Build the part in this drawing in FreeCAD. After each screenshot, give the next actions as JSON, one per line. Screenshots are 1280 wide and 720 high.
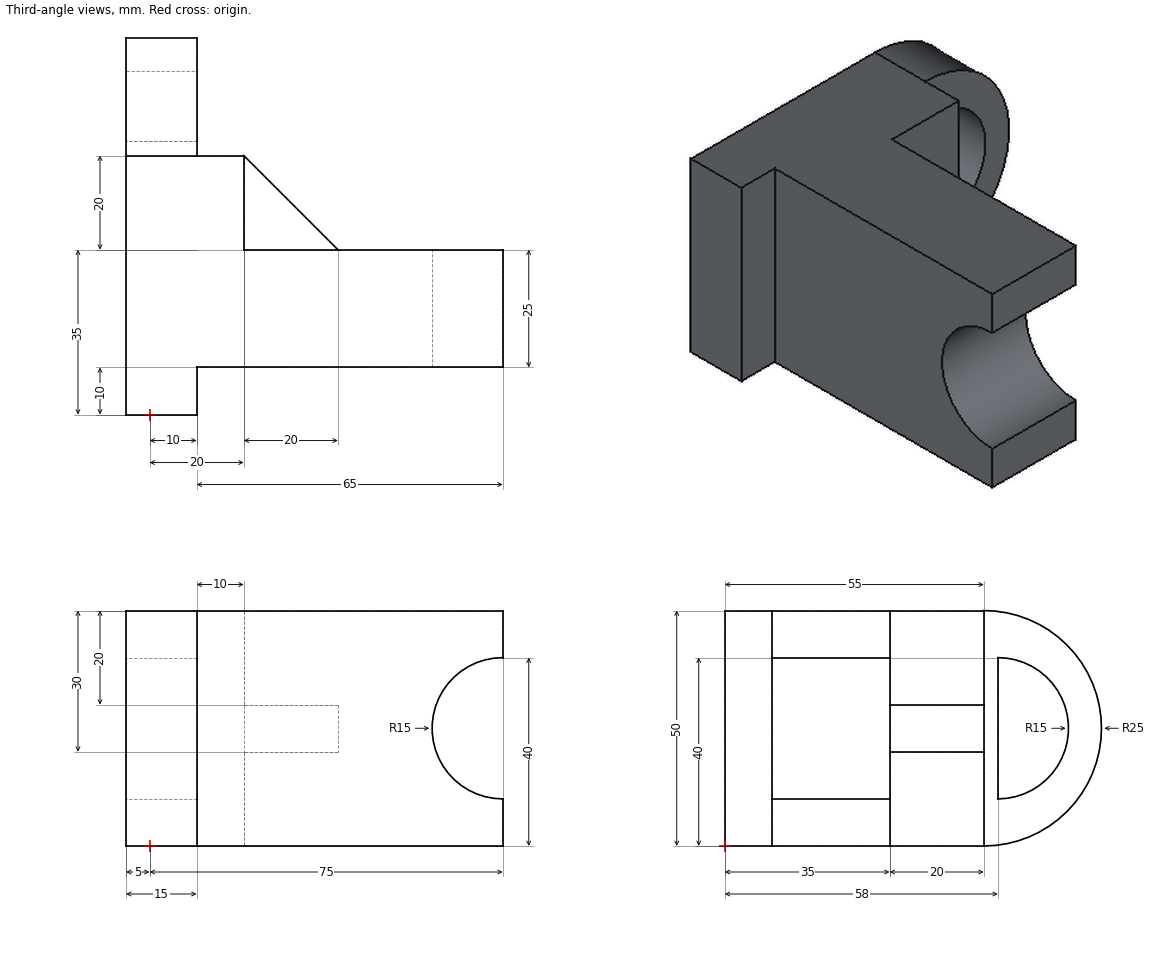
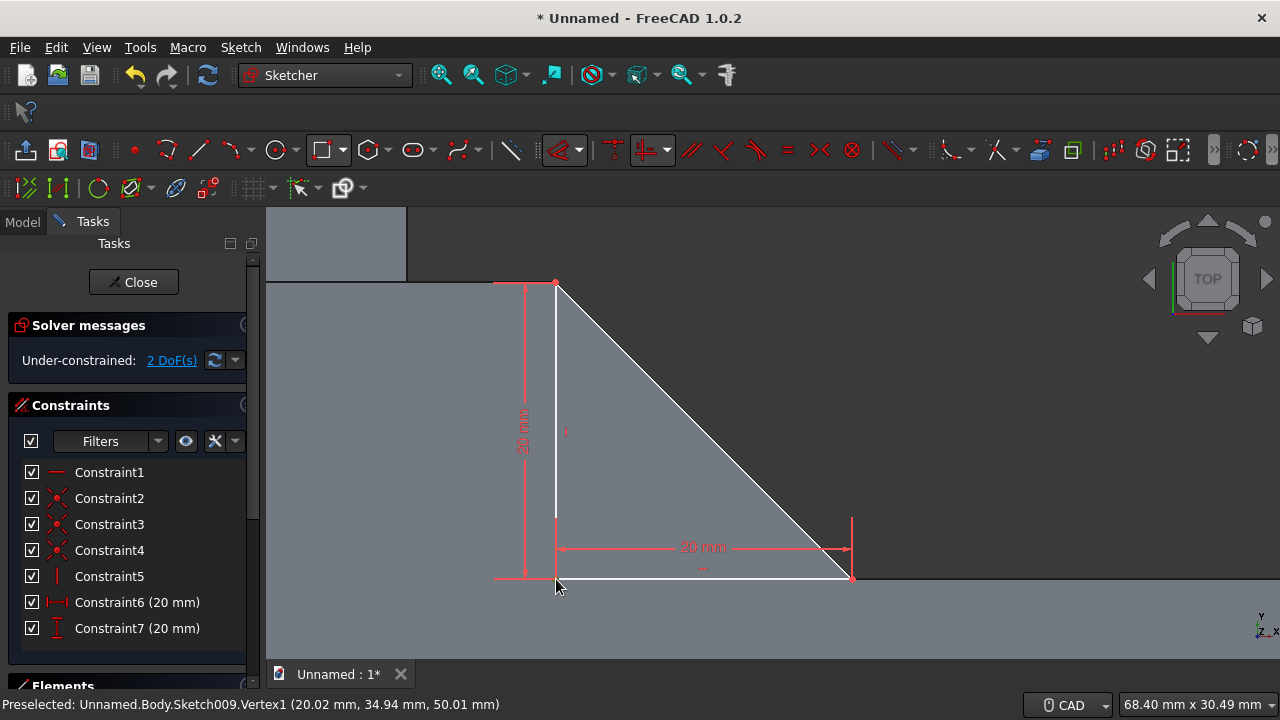
{"action": "key", "text": "l"}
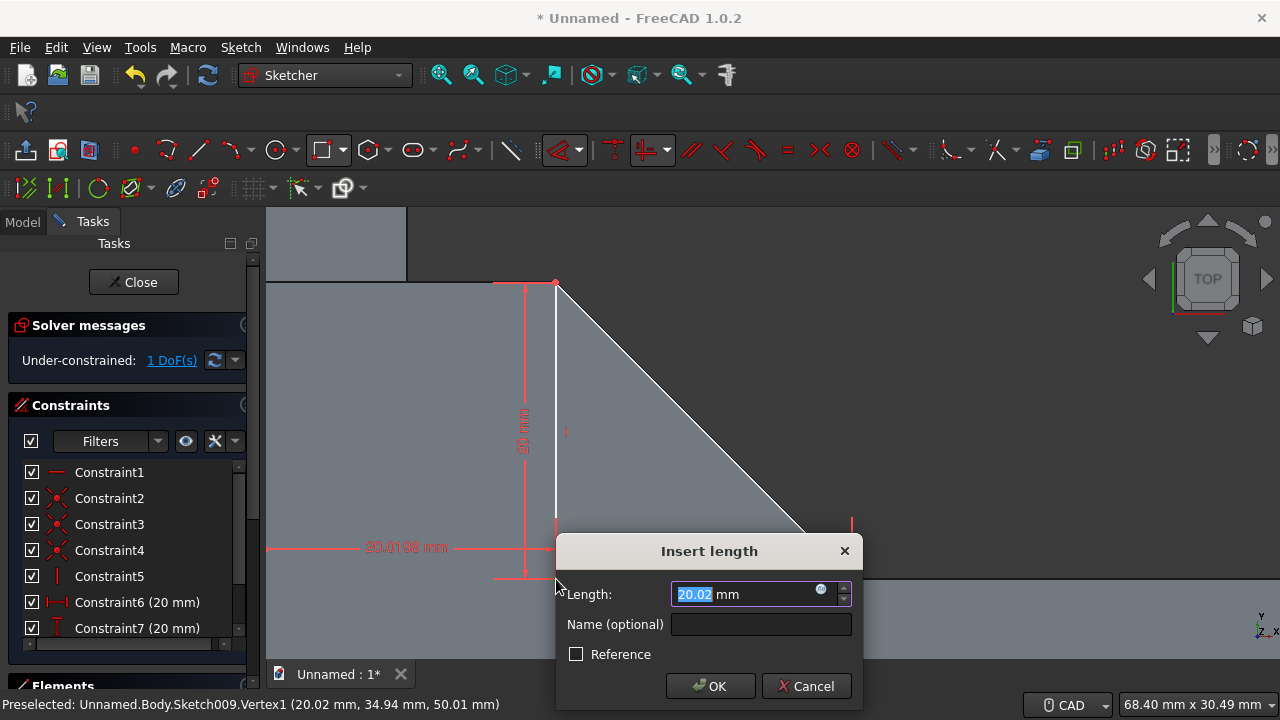
{"action": "type", "text": "20"}
{"action": "key", "text": "Return"}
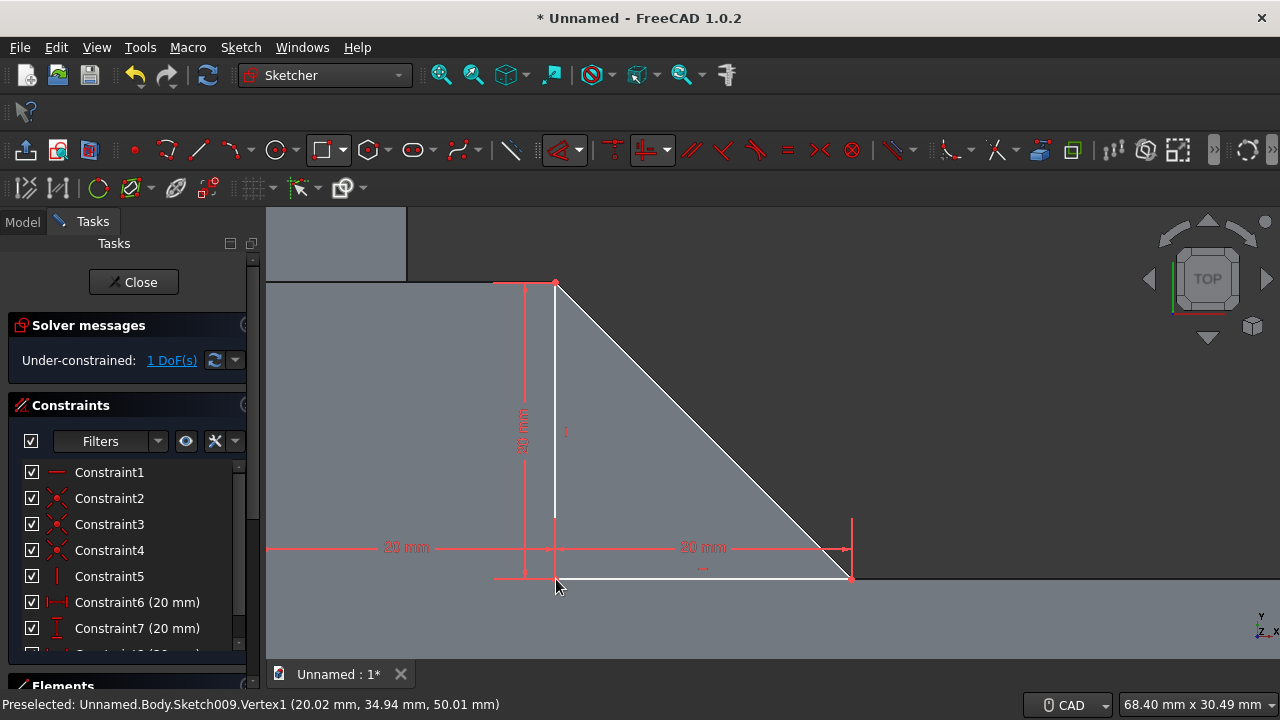
{"action": "left_click", "coordinate": [555, 579]}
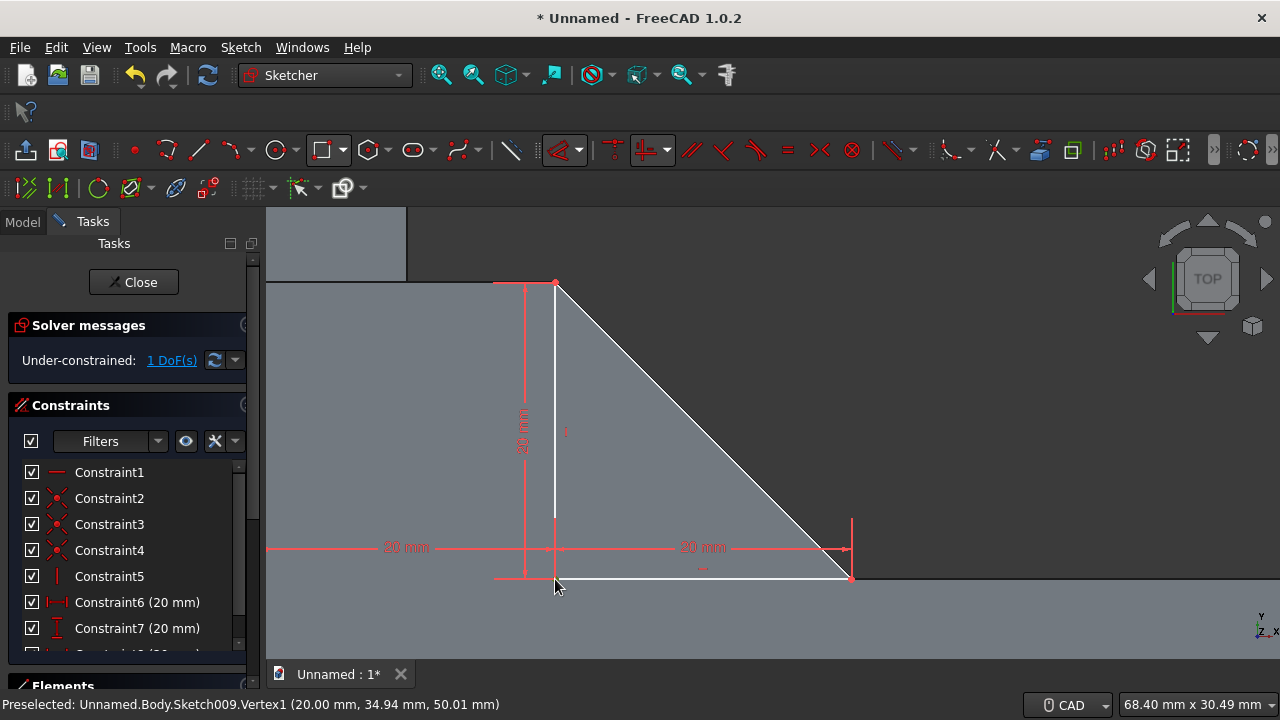
{"action": "left_click", "coordinate": [582, 150]}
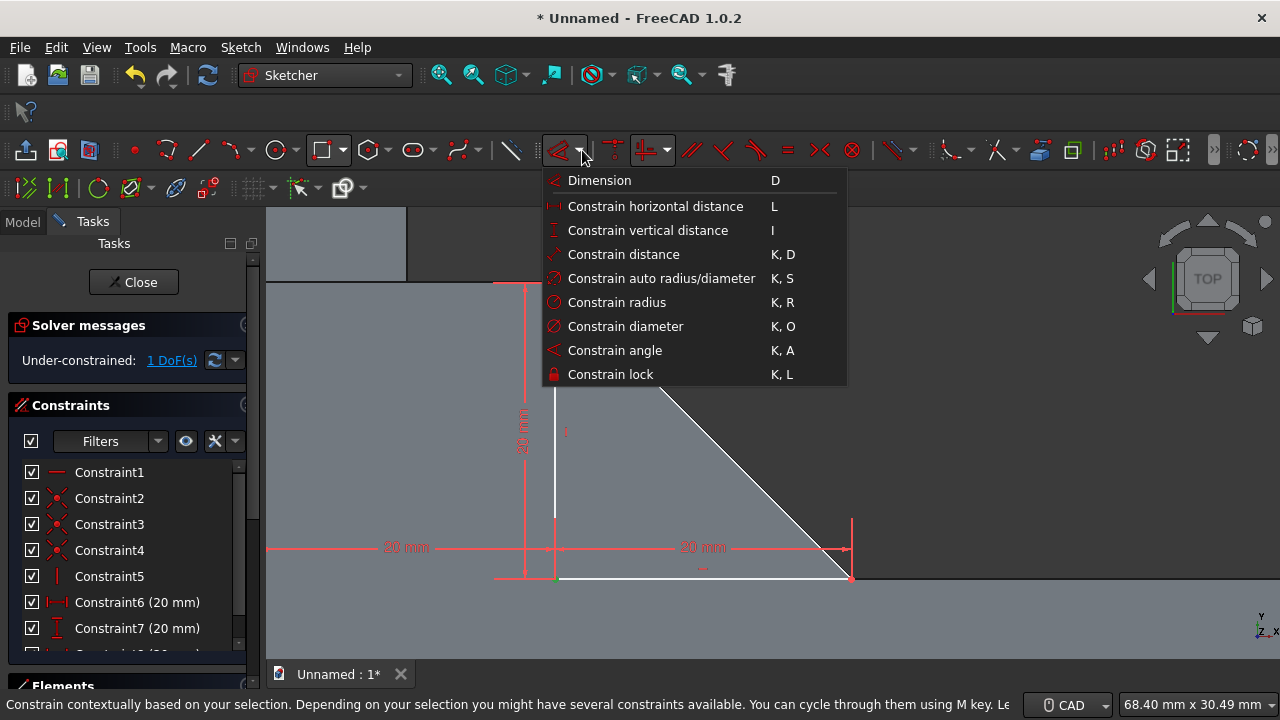
{"action": "left_click", "coordinate": [695, 230]}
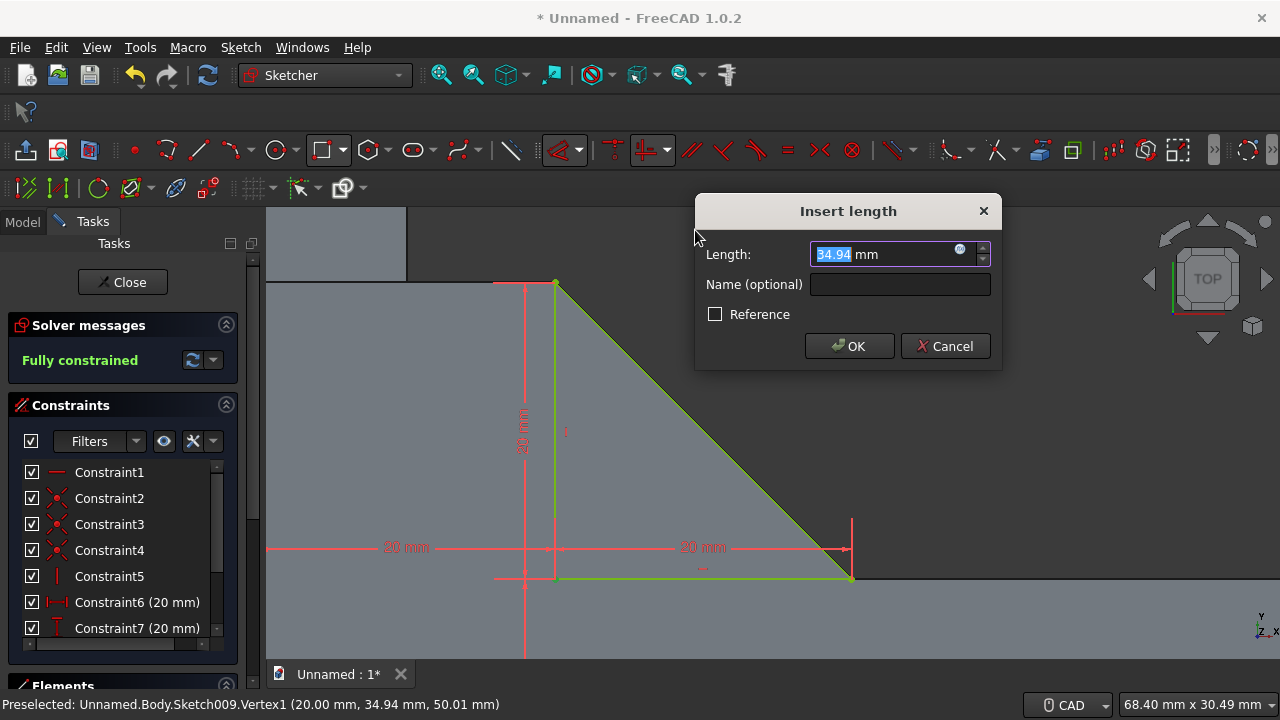
{"action": "type", "text": "35"}
{"action": "key", "text": "Return"}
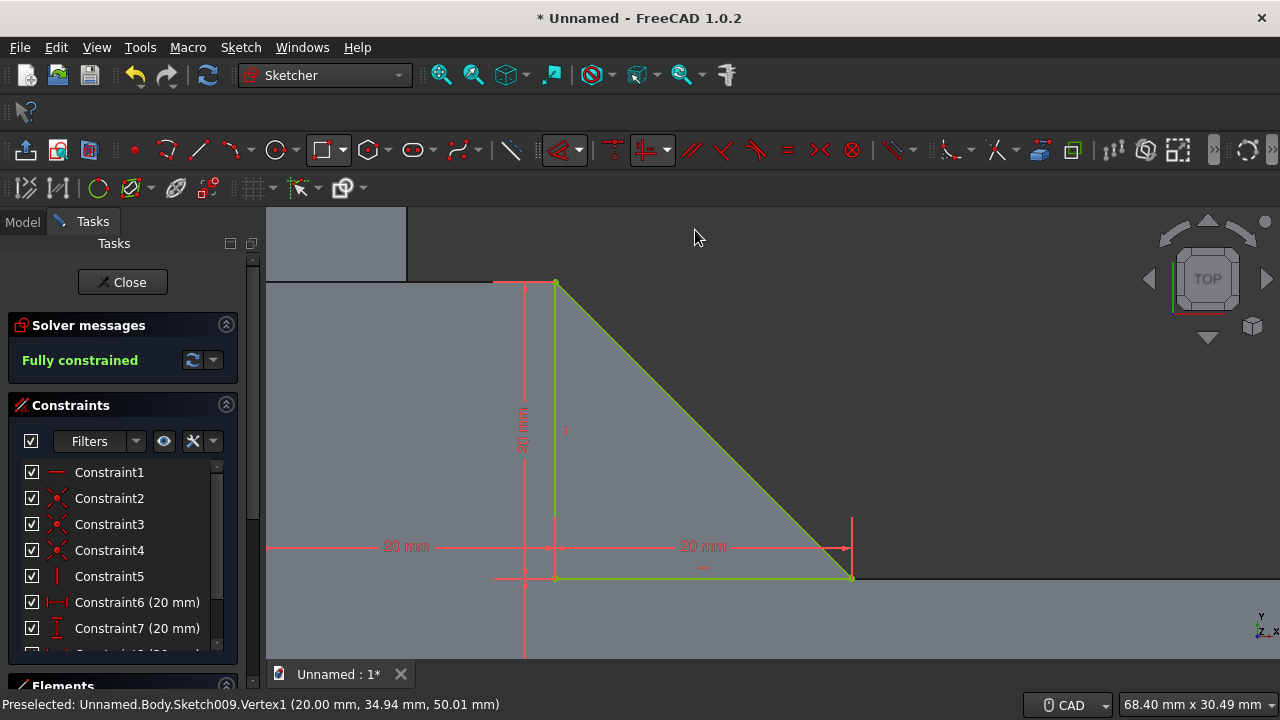
{"action": "left_click", "coordinate": [123, 282]}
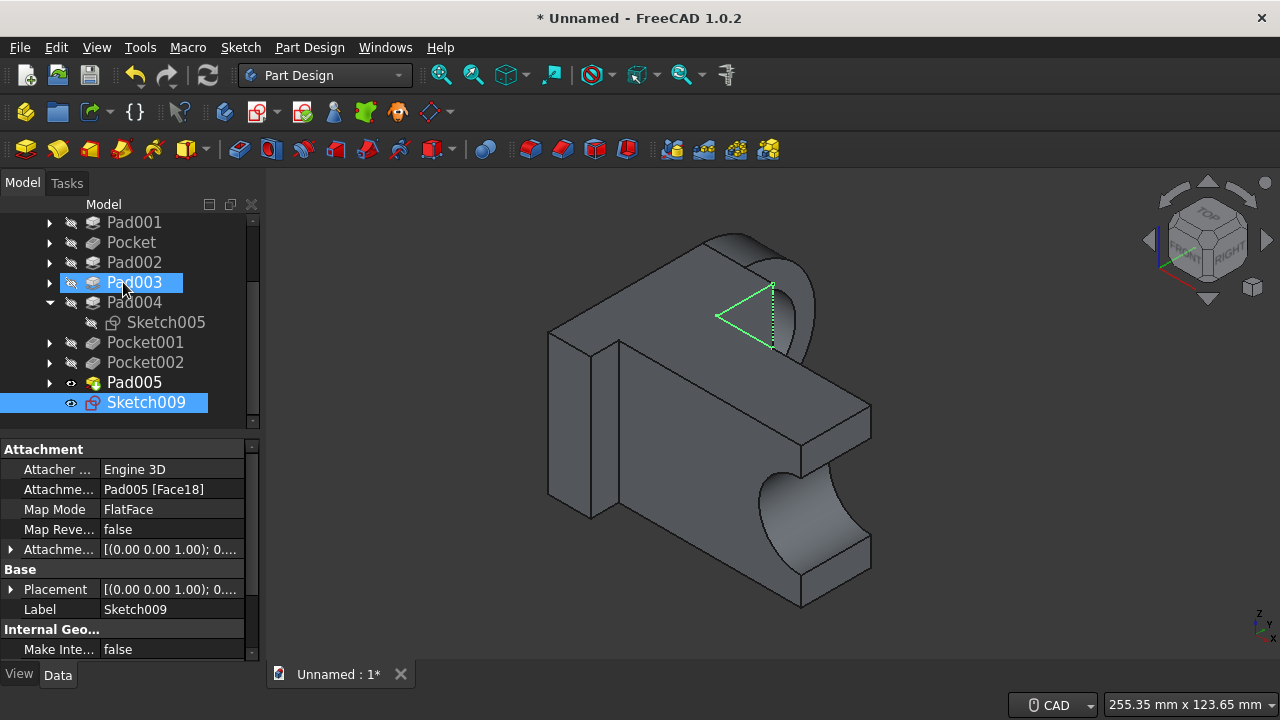
{"action": "left_click", "coordinate": [240, 150]}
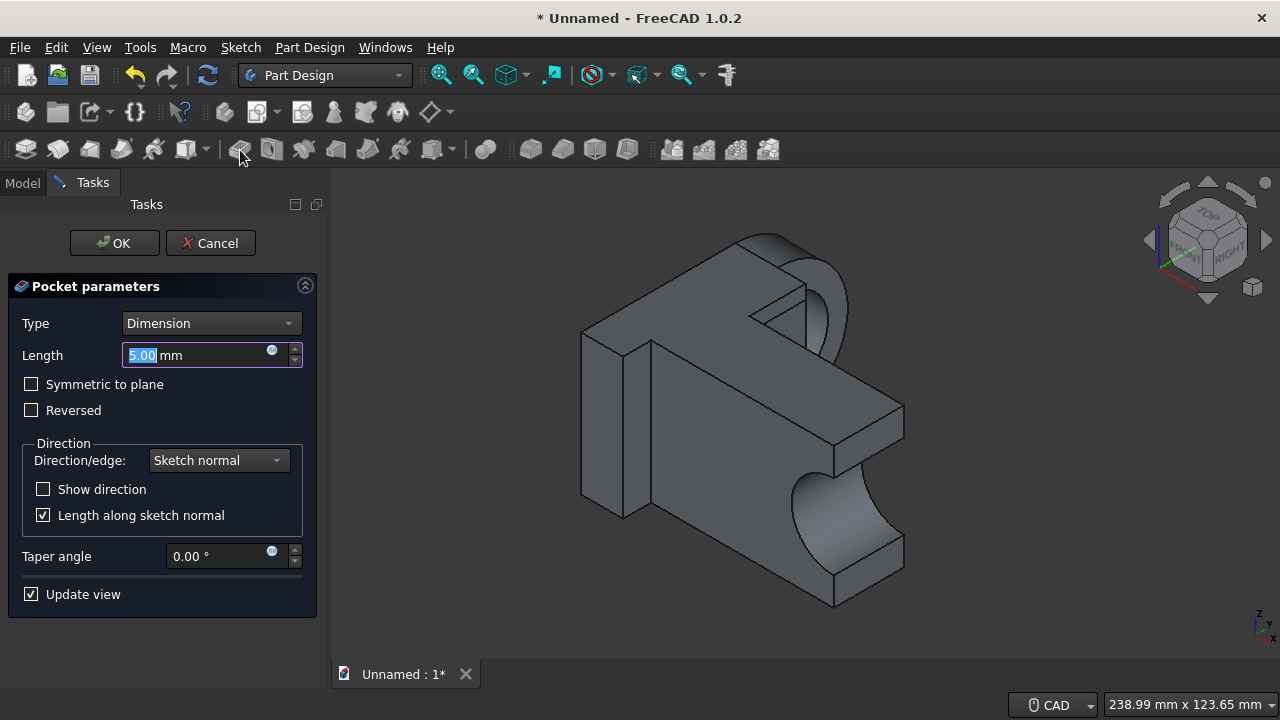
{"action": "type", "text": "20"}
{"action": "key", "text": "Tab"}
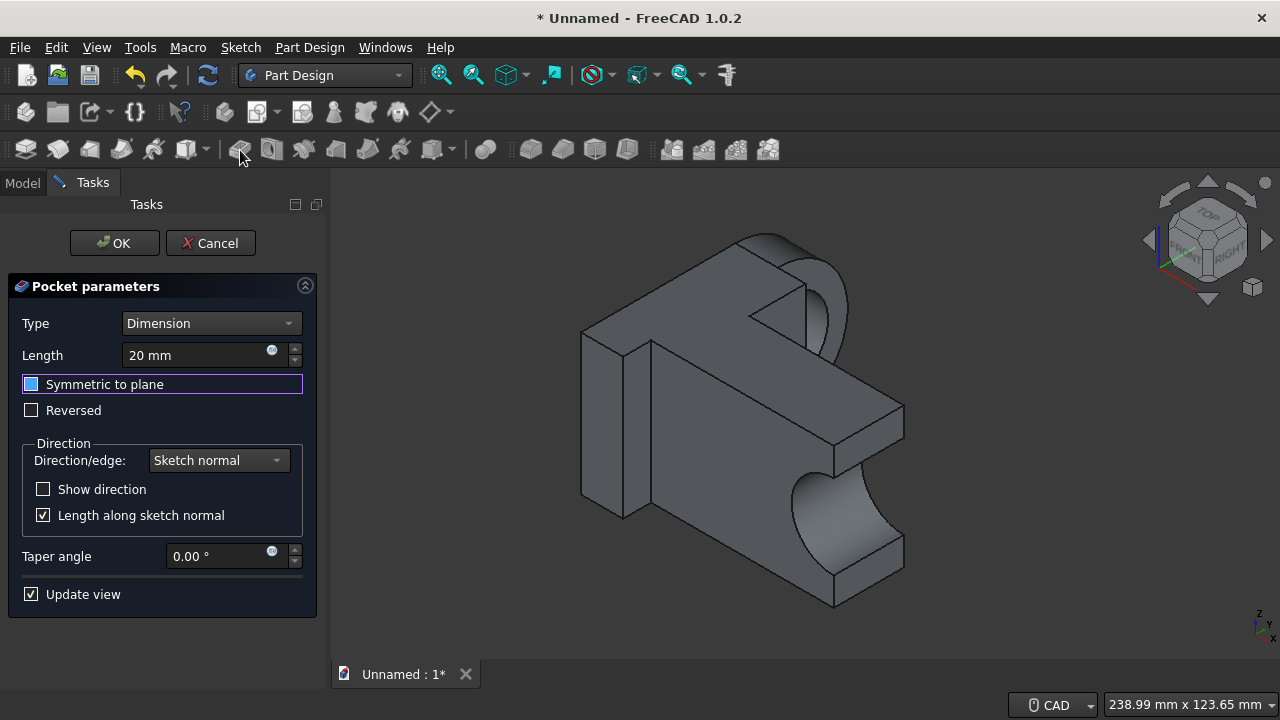
{"action": "left_click", "coordinate": [115, 243]}